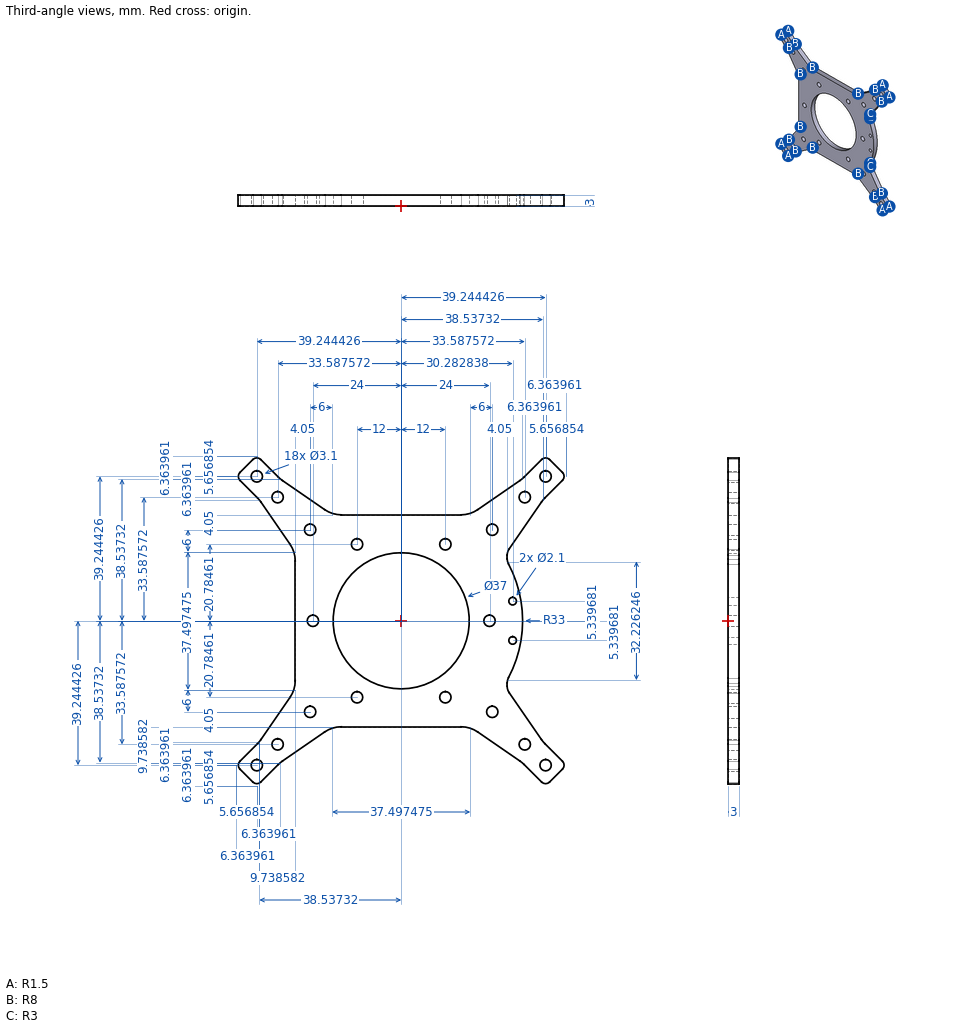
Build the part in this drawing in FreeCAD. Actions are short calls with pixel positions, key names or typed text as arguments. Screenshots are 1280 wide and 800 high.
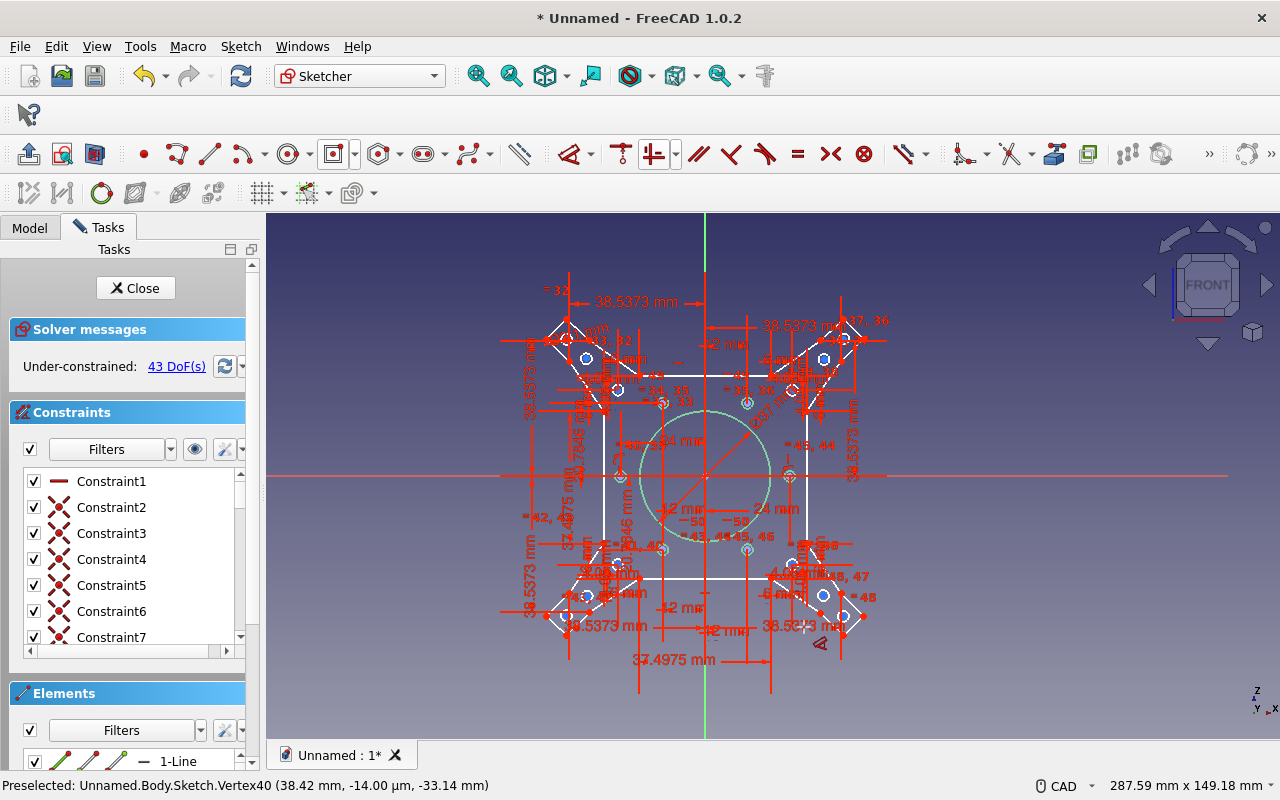
click(821, 613)
click(855, 513)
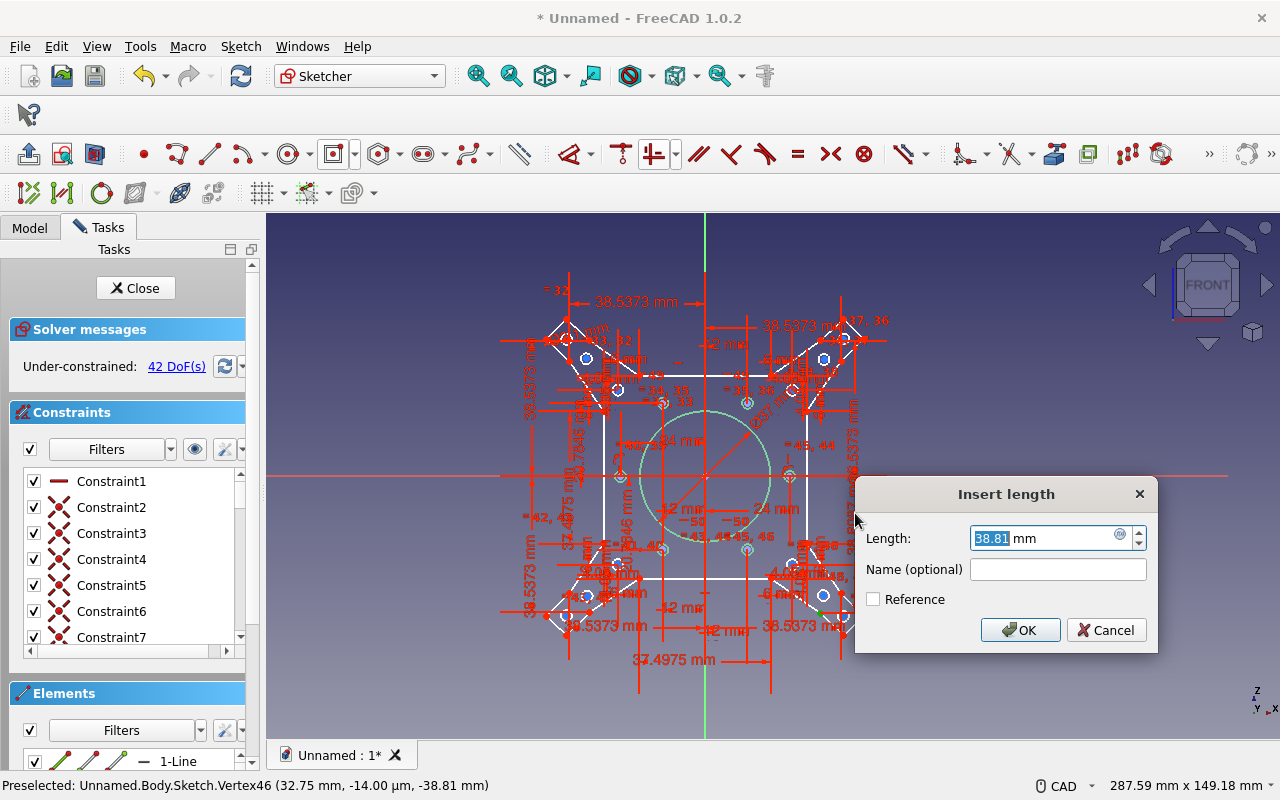
text(38.53732)
key(Return)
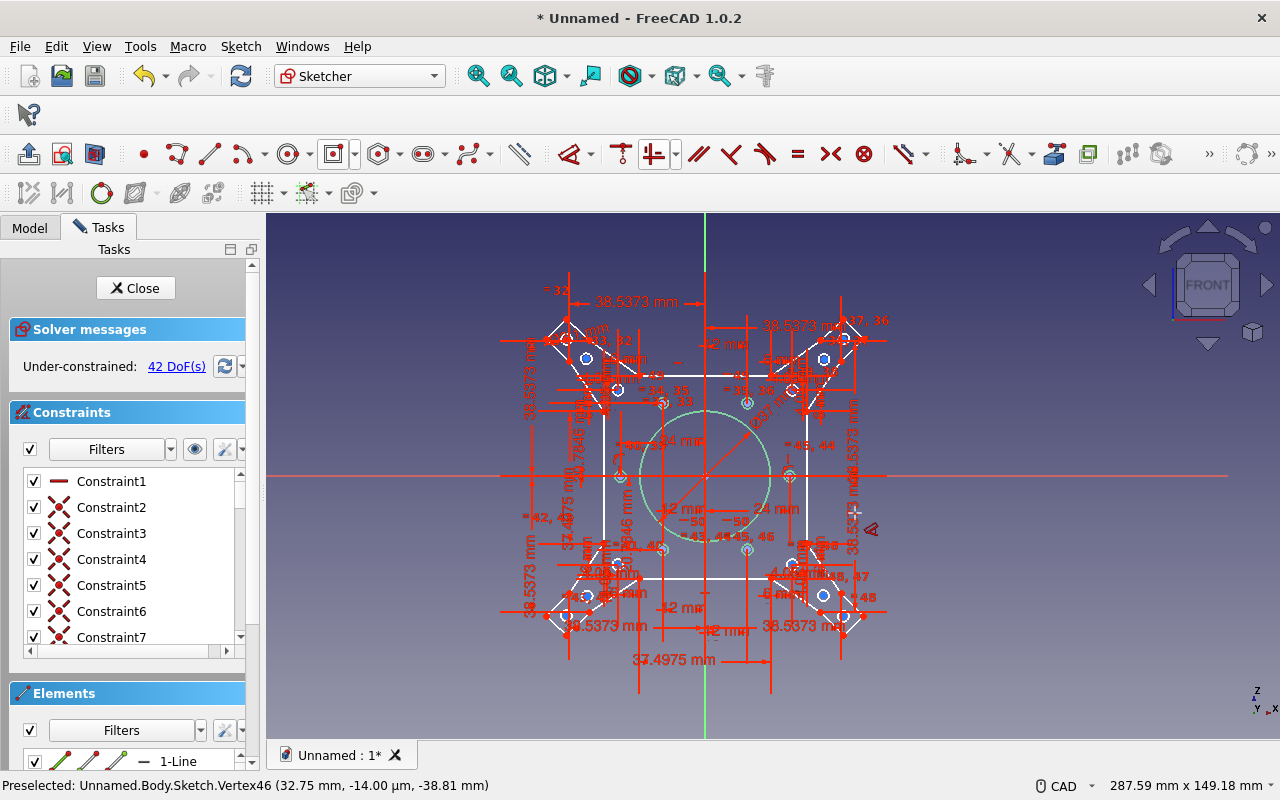
click(624, 589)
click(532, 603)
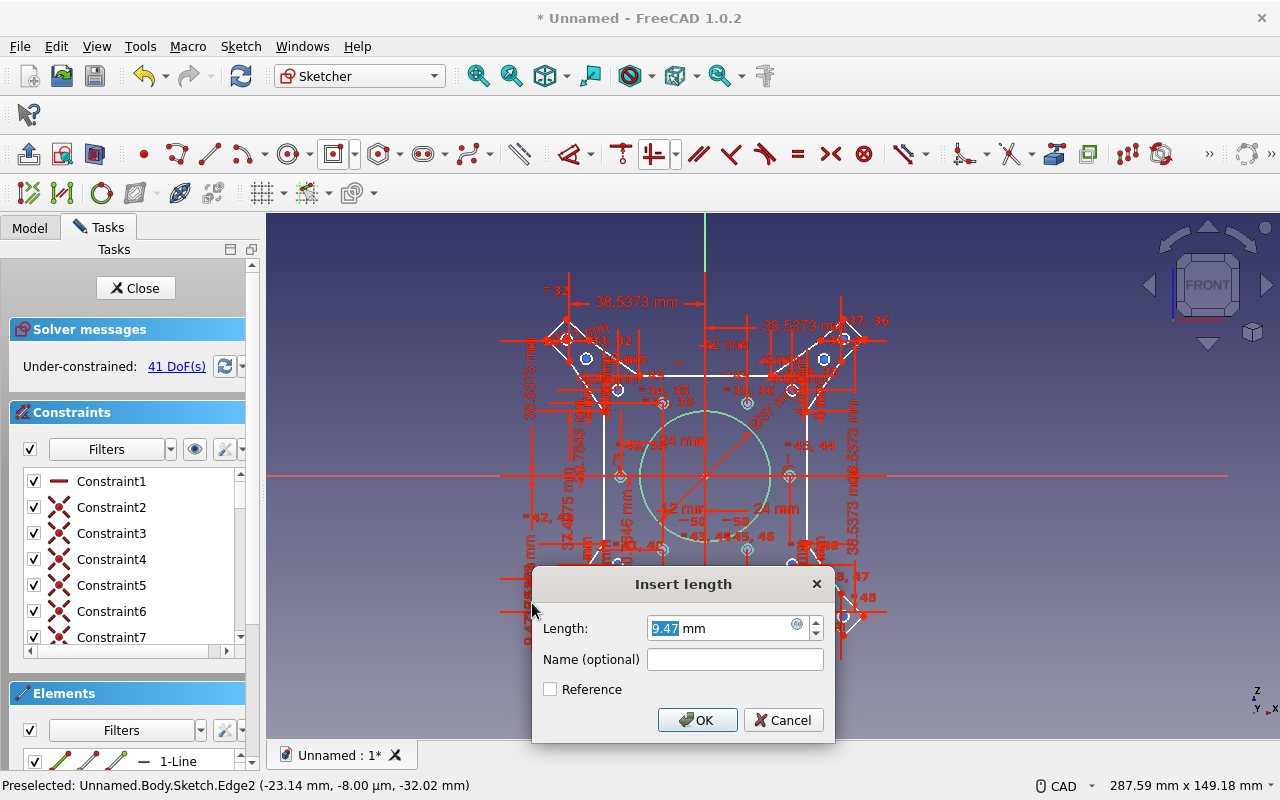
text(9.738582)
key(Return)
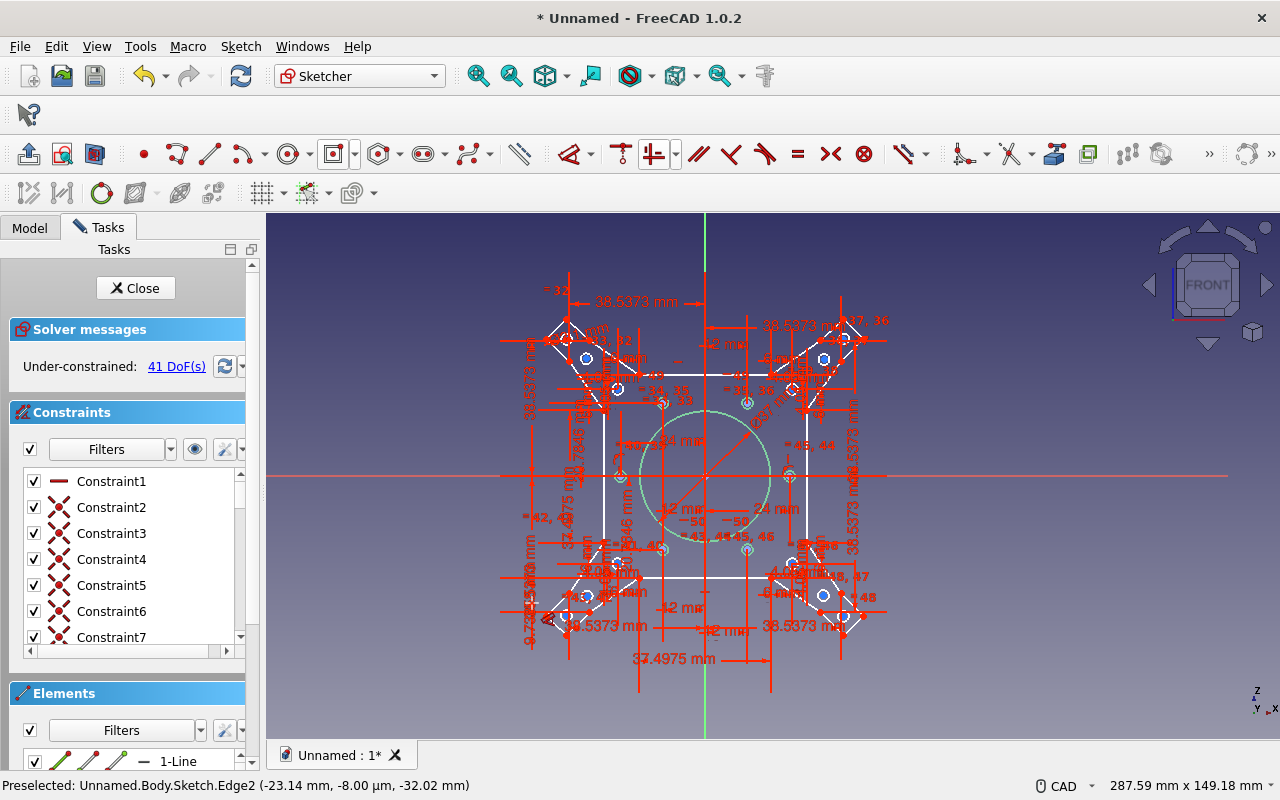
scroll(583, 619, up, 3)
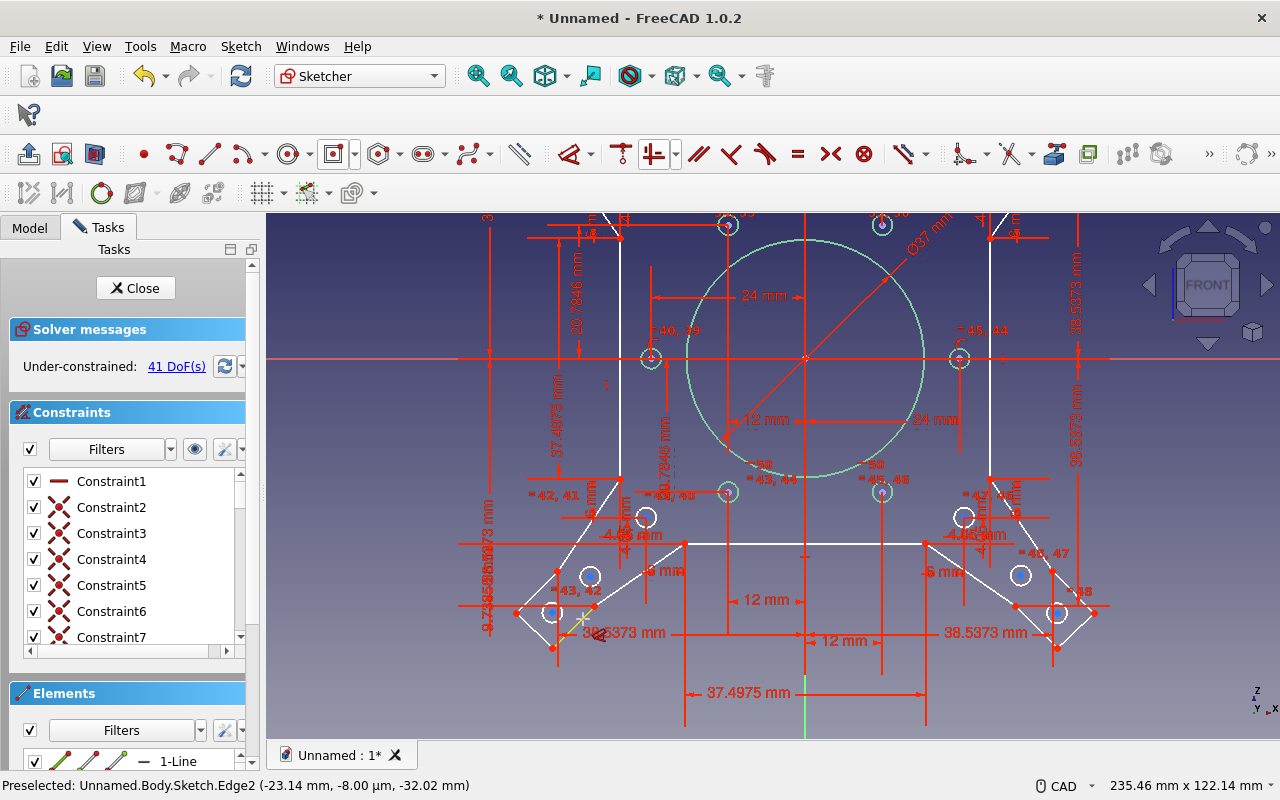
click(582, 619)
click(574, 682)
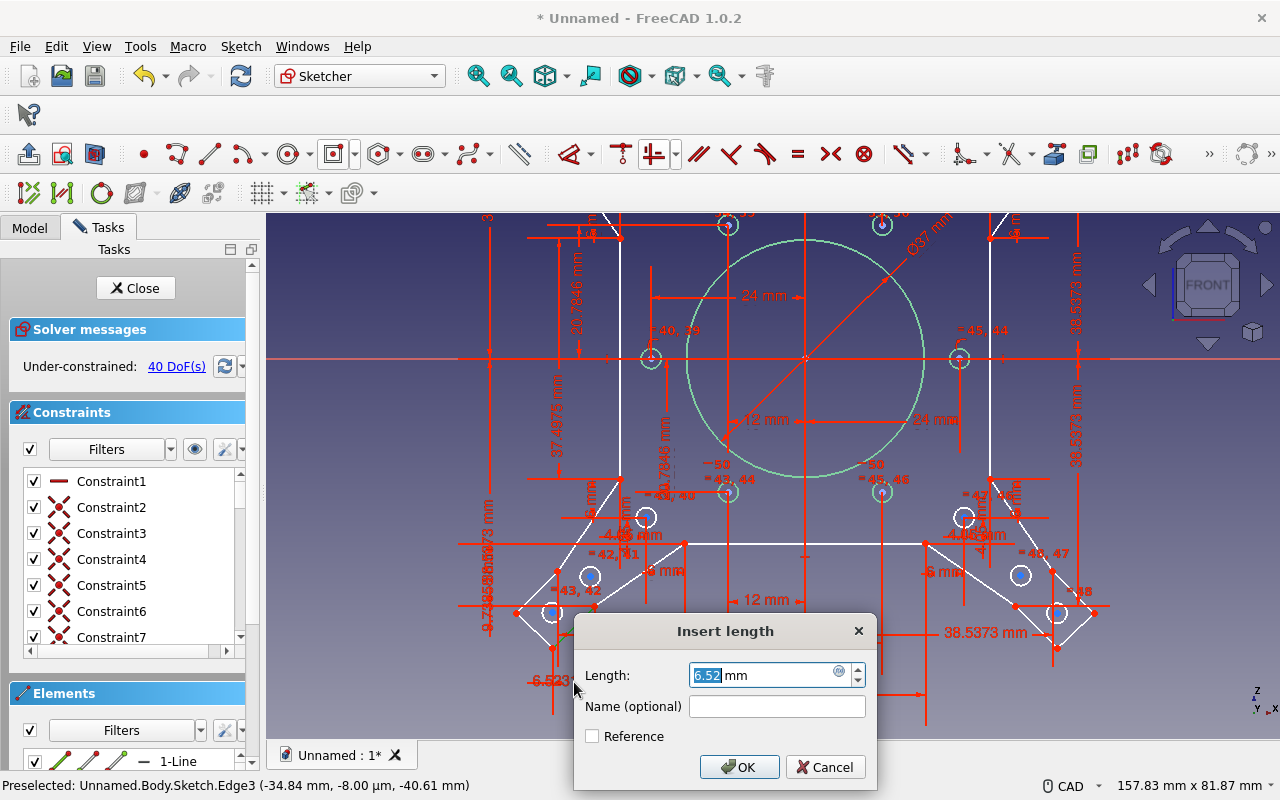
text(6.363961)
key(Return)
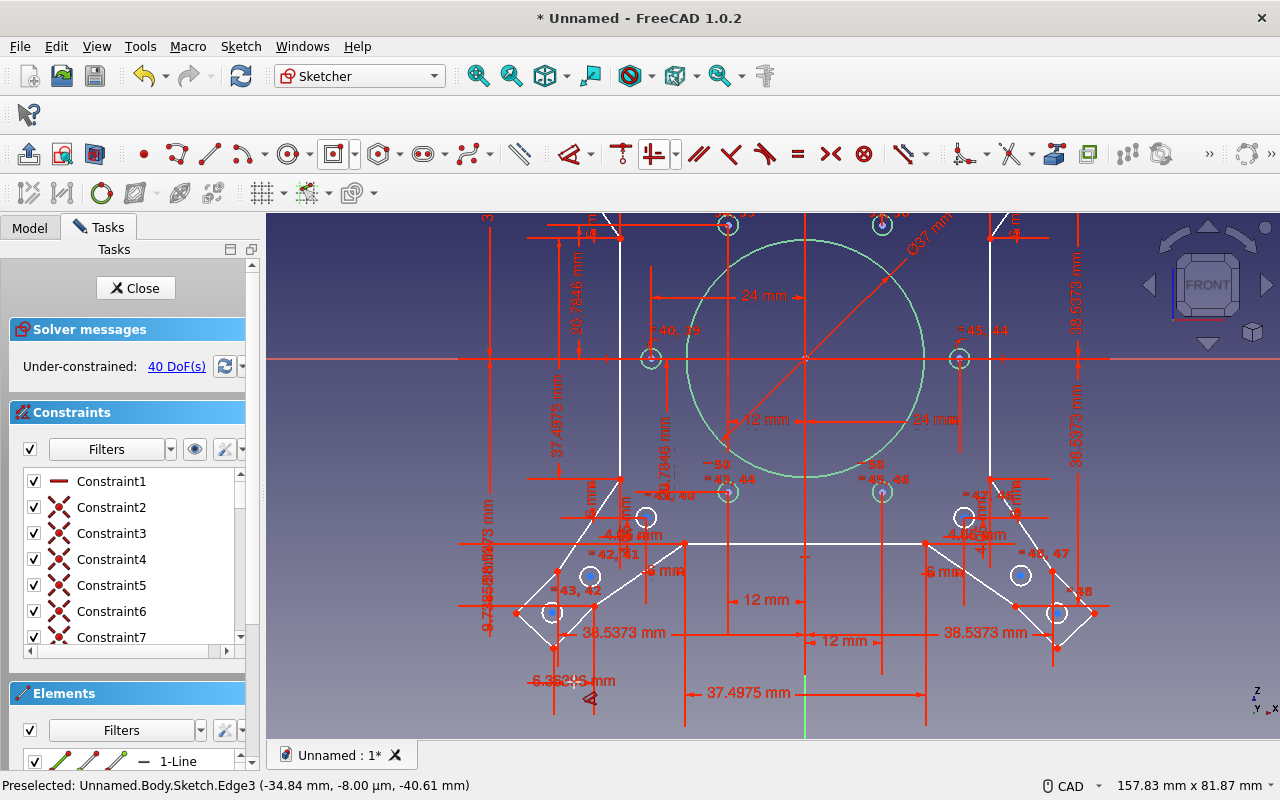
click(582, 619)
click(520, 637)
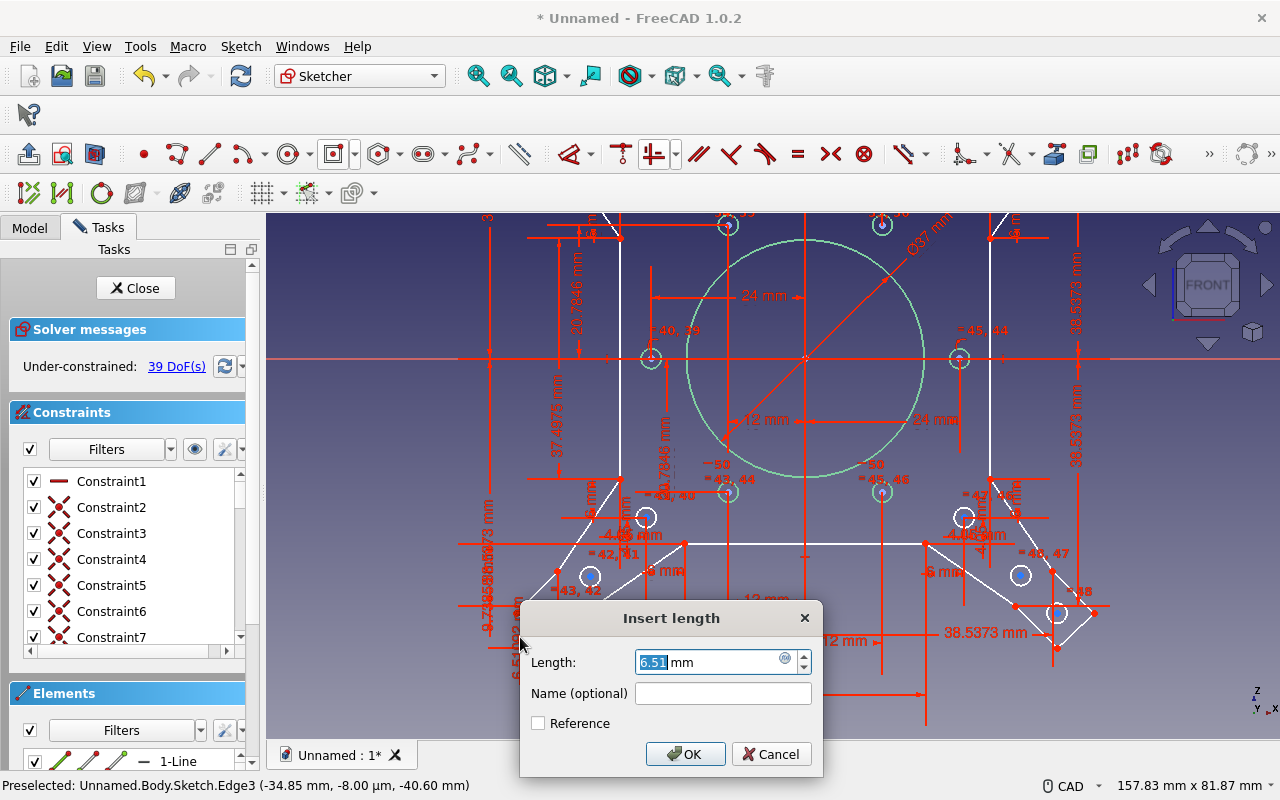
text(6.363961)
key(Return)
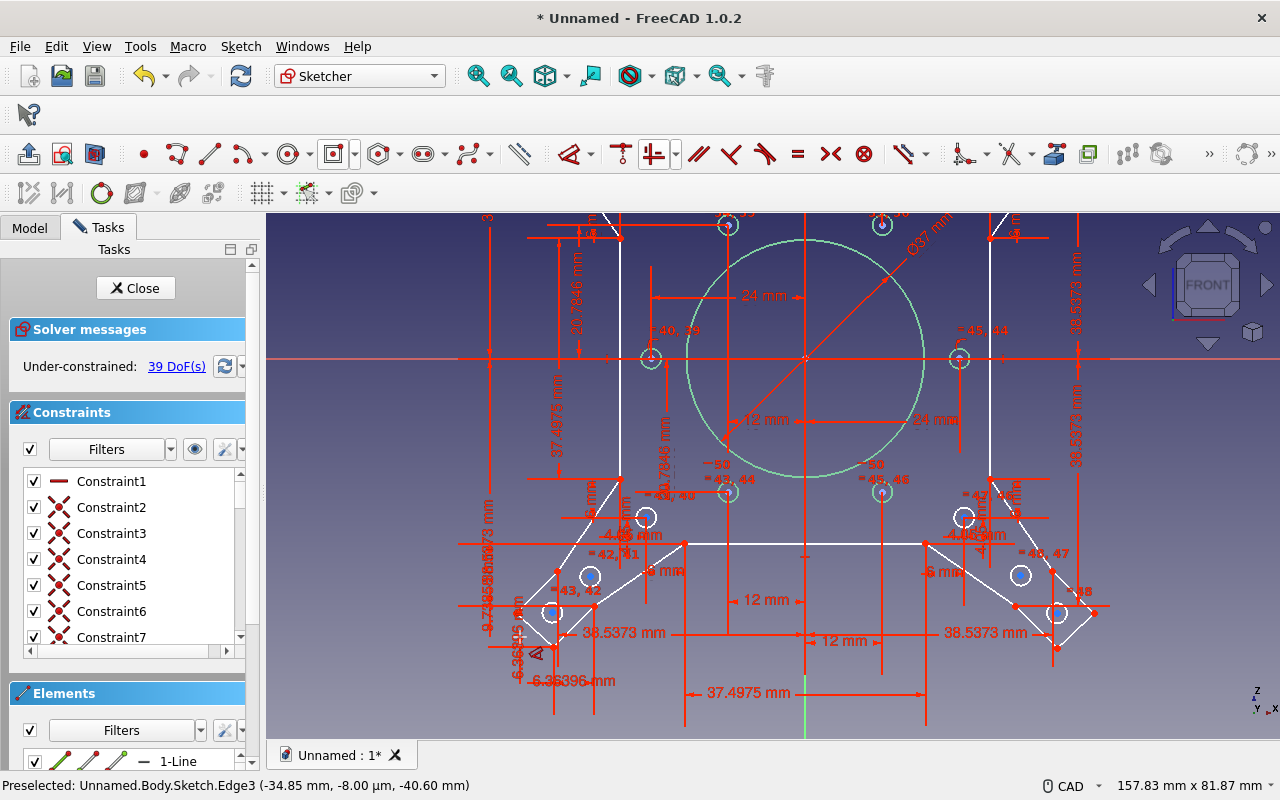
click(542, 637)
click(535, 705)